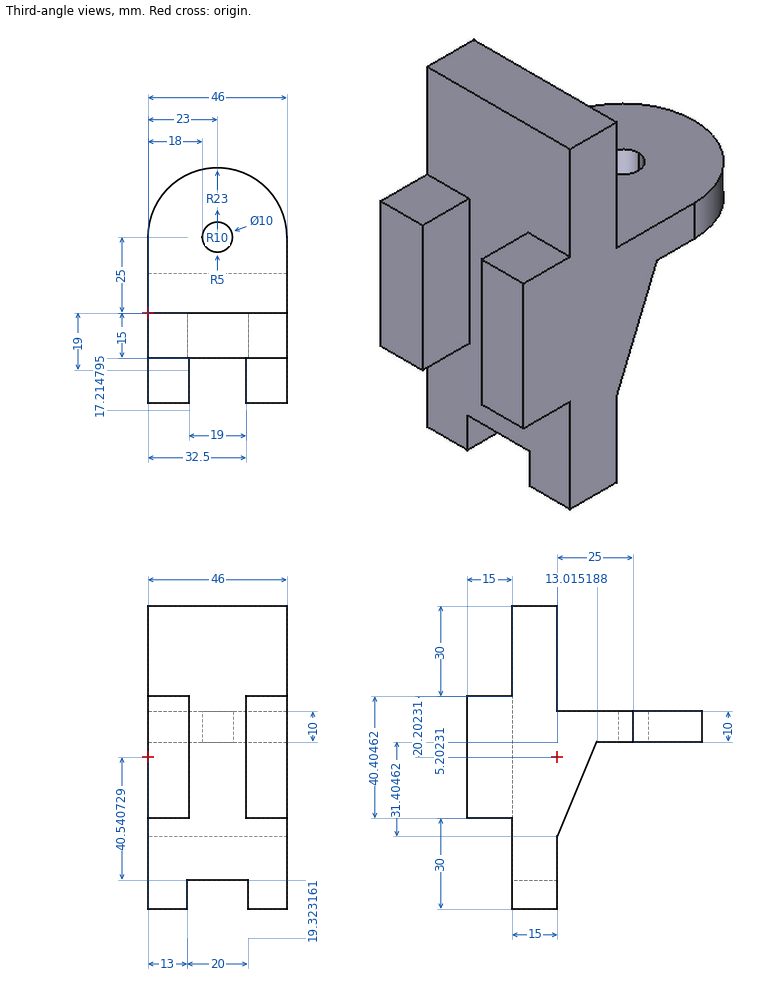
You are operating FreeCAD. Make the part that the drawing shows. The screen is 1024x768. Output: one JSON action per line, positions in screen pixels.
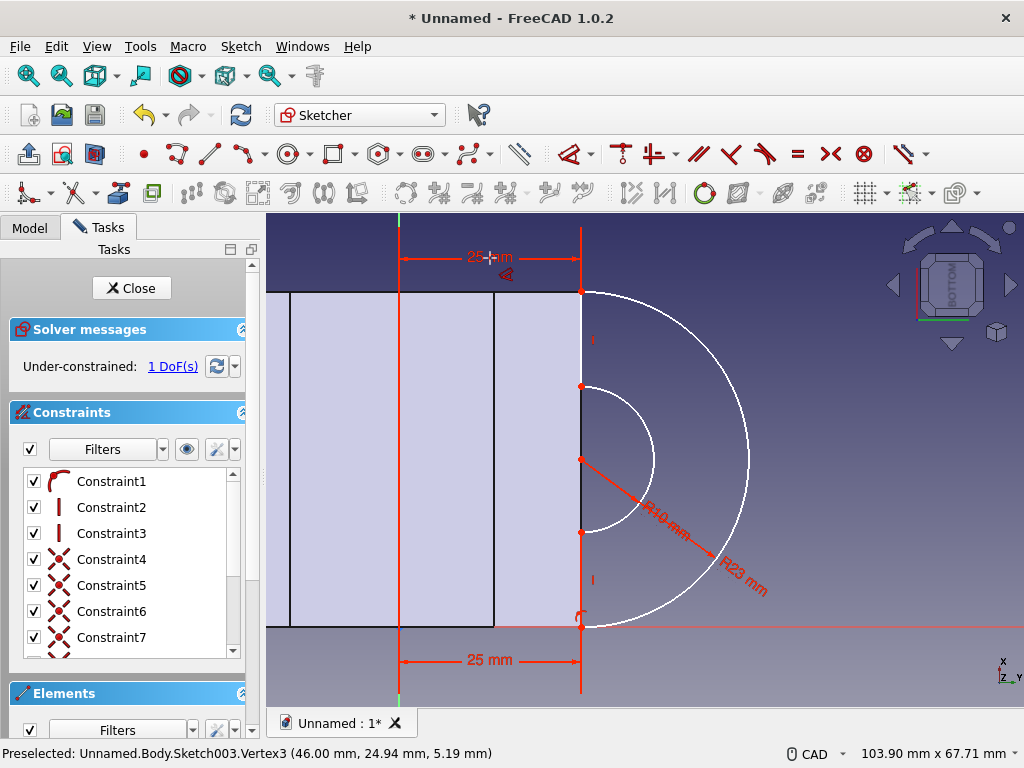
{"action": "left_click", "coordinate": [581, 460]}
{"action": "left_click", "coordinate": [490, 426]}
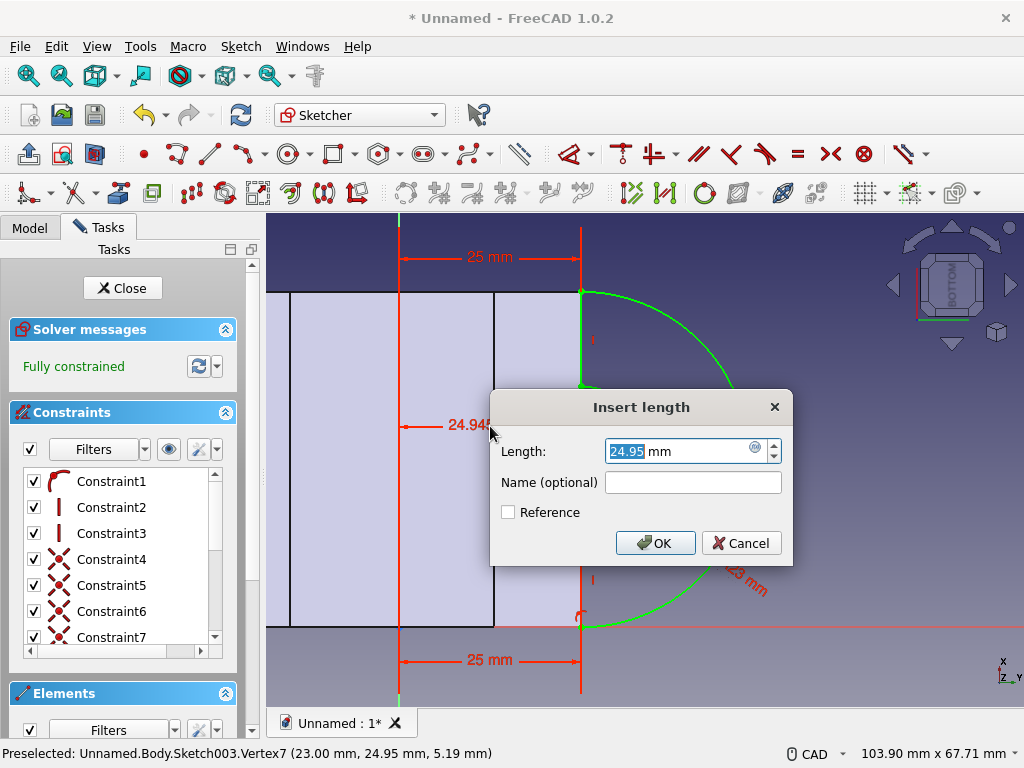
{"action": "type", "text": "25"}
{"action": "key", "text": "Return"}
{"action": "key", "text": "Escape"}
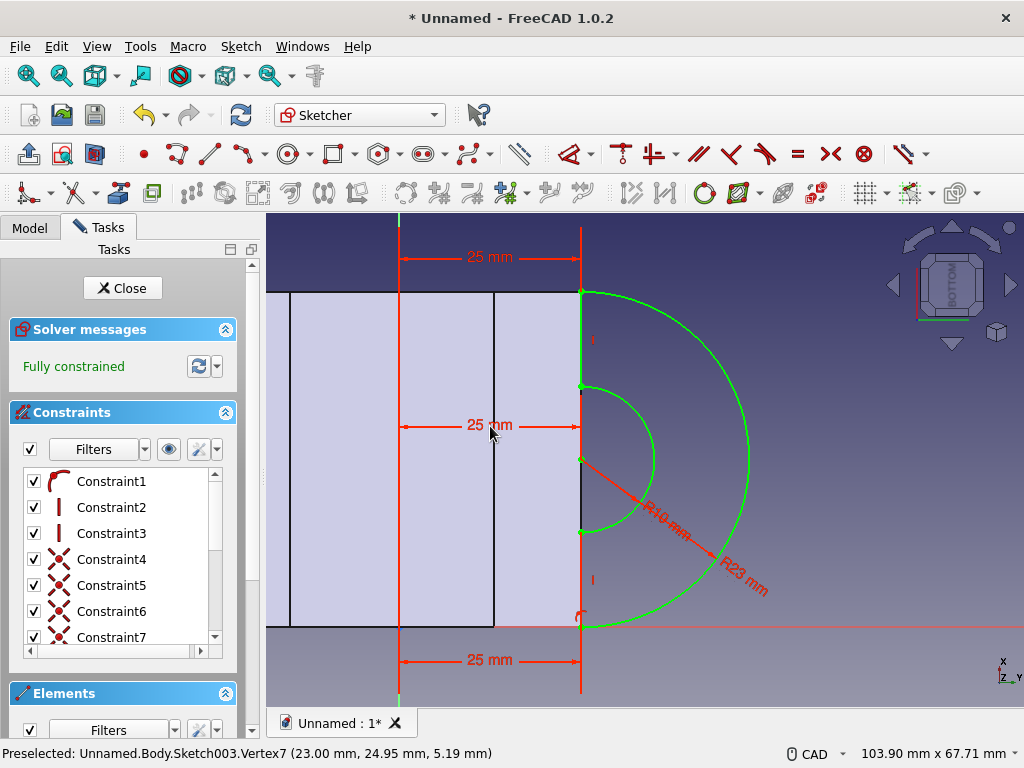
{"action": "left_click", "coordinate": [123, 288]}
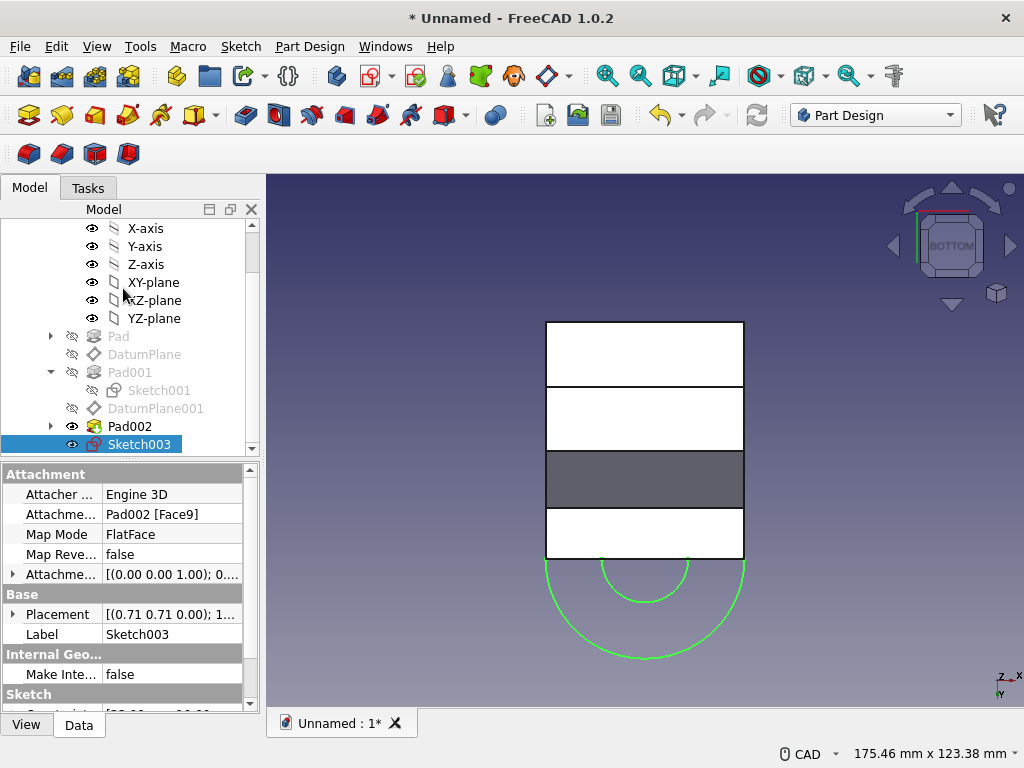
{"action": "left_click", "coordinate": [29, 116]}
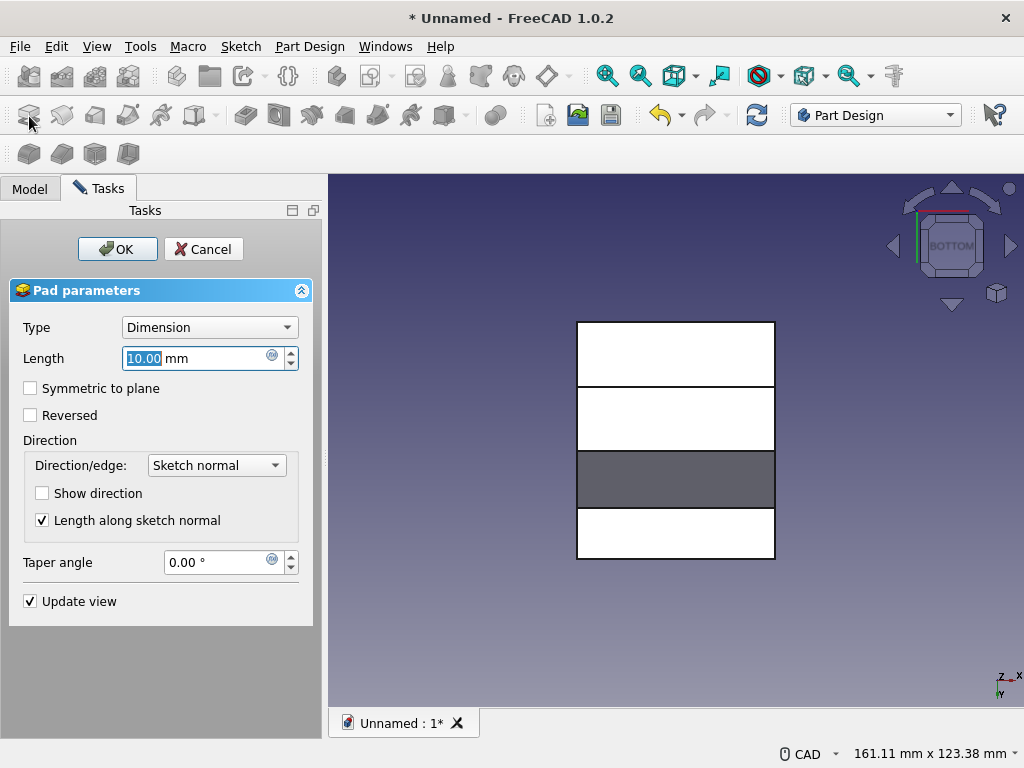
{"action": "type", "text": "10"}
{"action": "key", "text": "Tab"}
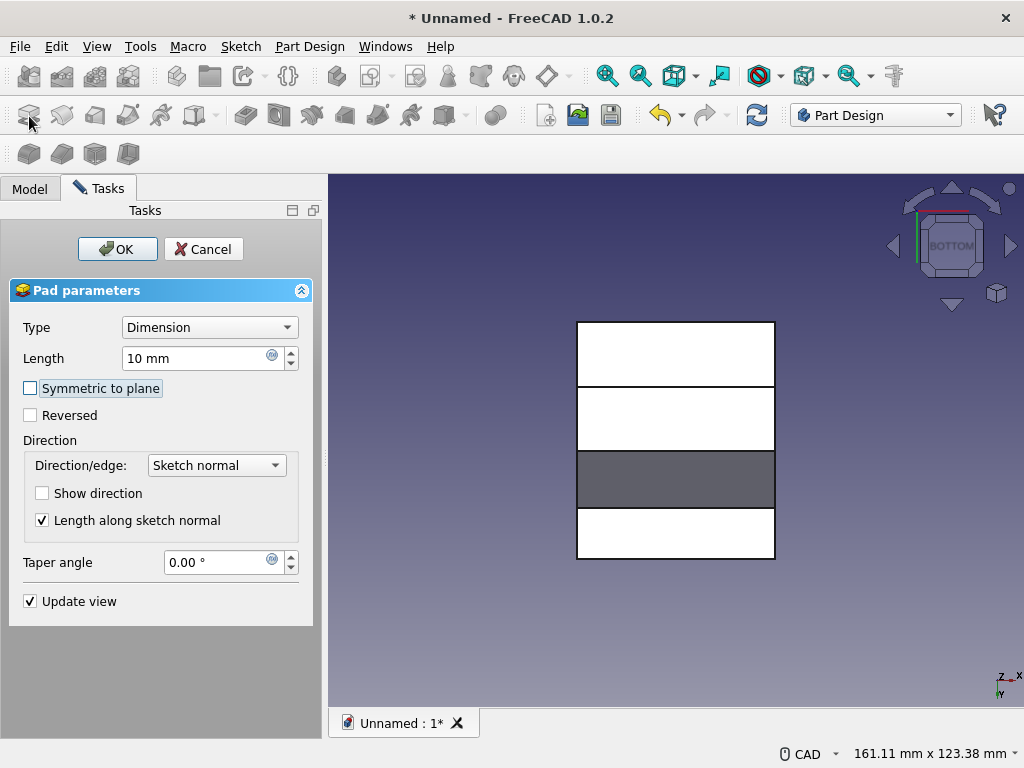
{"action": "left_click", "coordinate": [31, 415]}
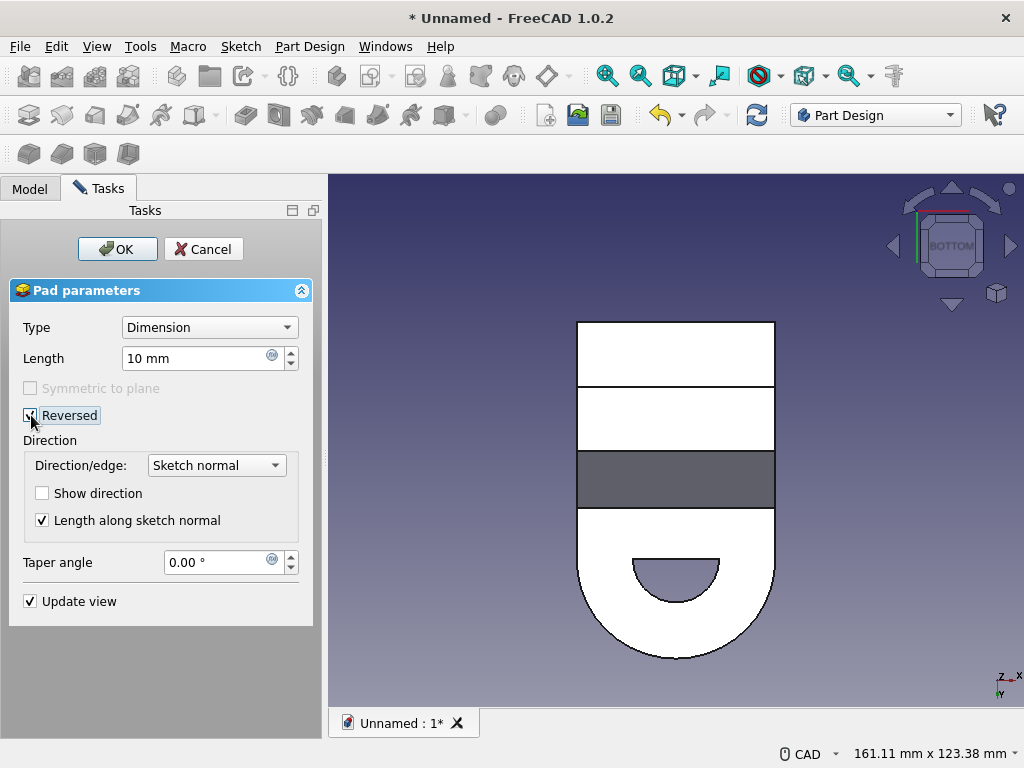
{"action": "left_click", "coordinate": [118, 249]}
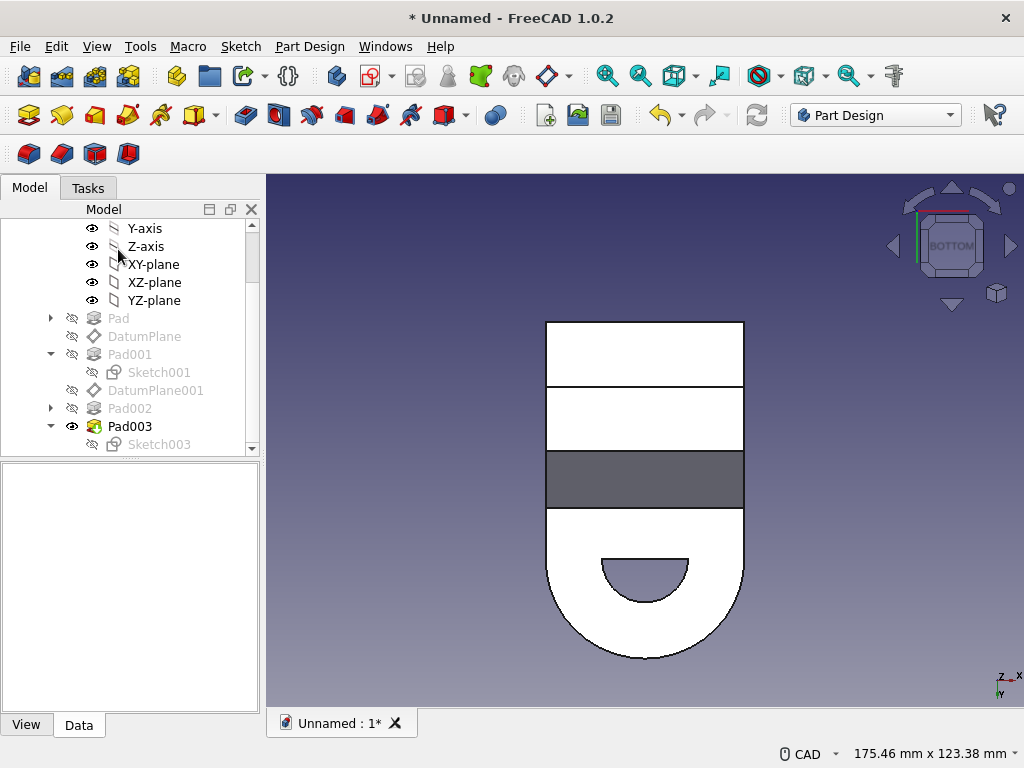
{"action": "left_click", "coordinate": [588, 604]}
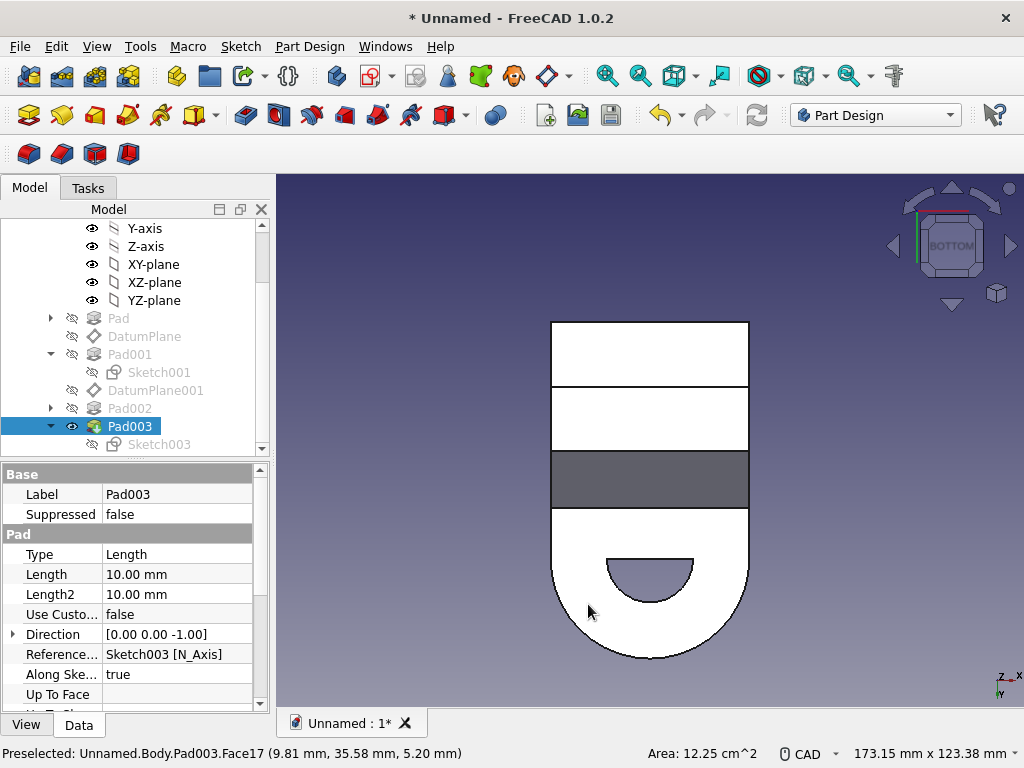
{"action": "left_click", "coordinate": [370, 76]}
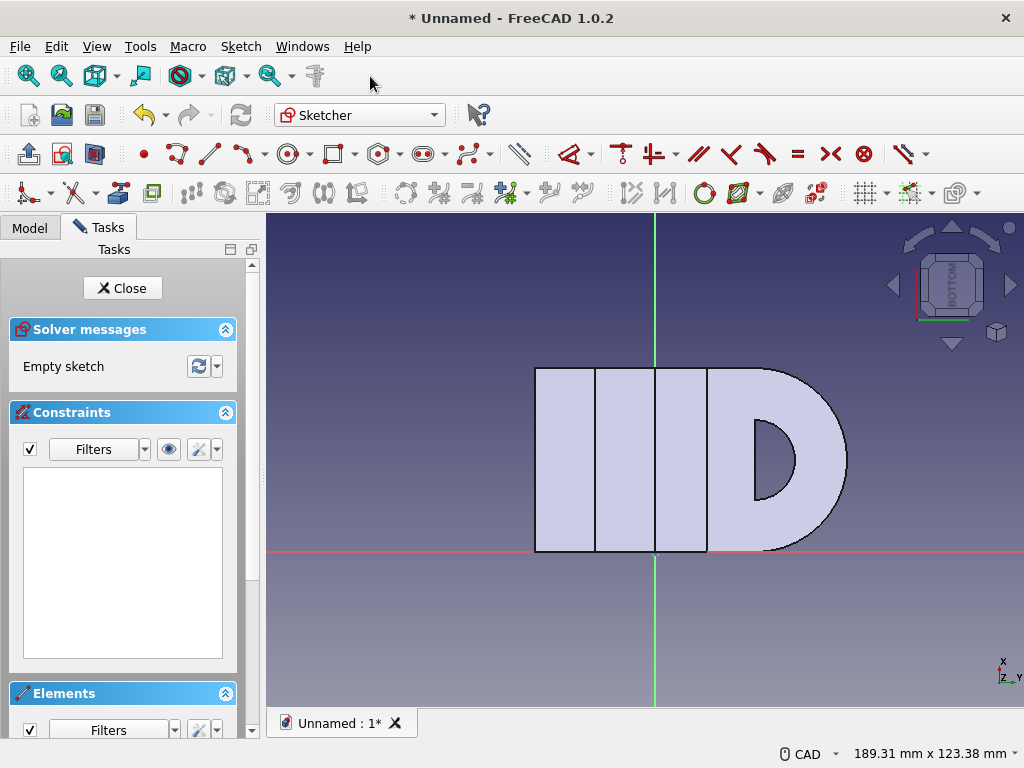
{"action": "scroll", "coordinate": [846, 507], "scroll_direction": "up", "scroll_amount": 4}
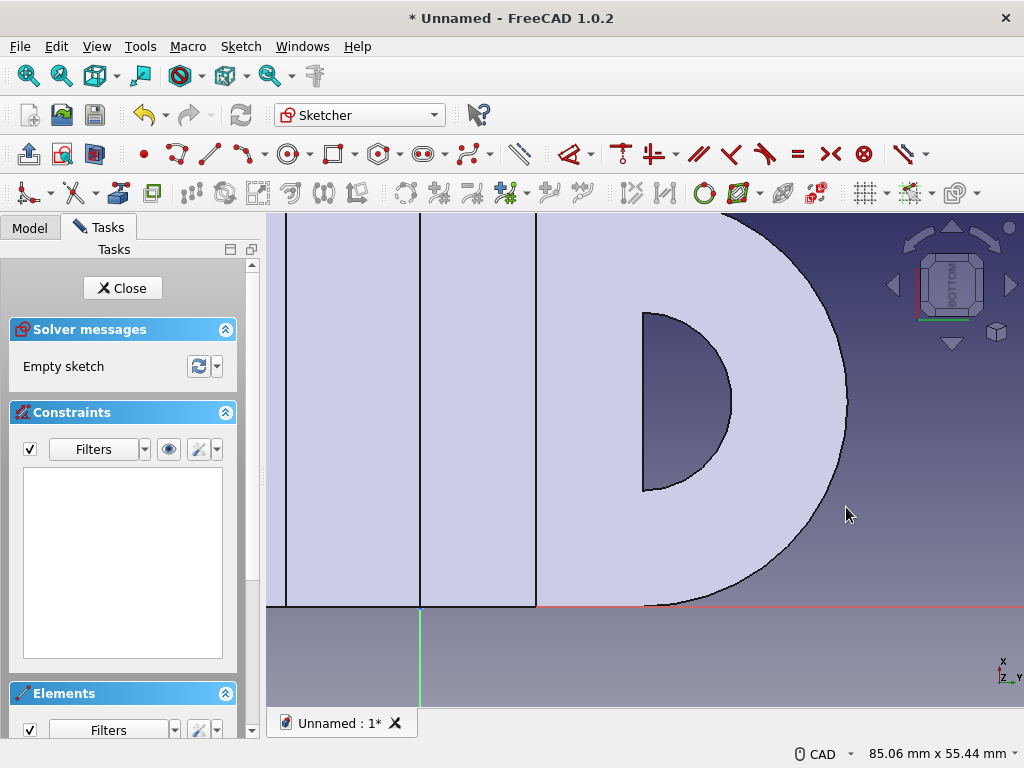
{"action": "key", "text": "g l"}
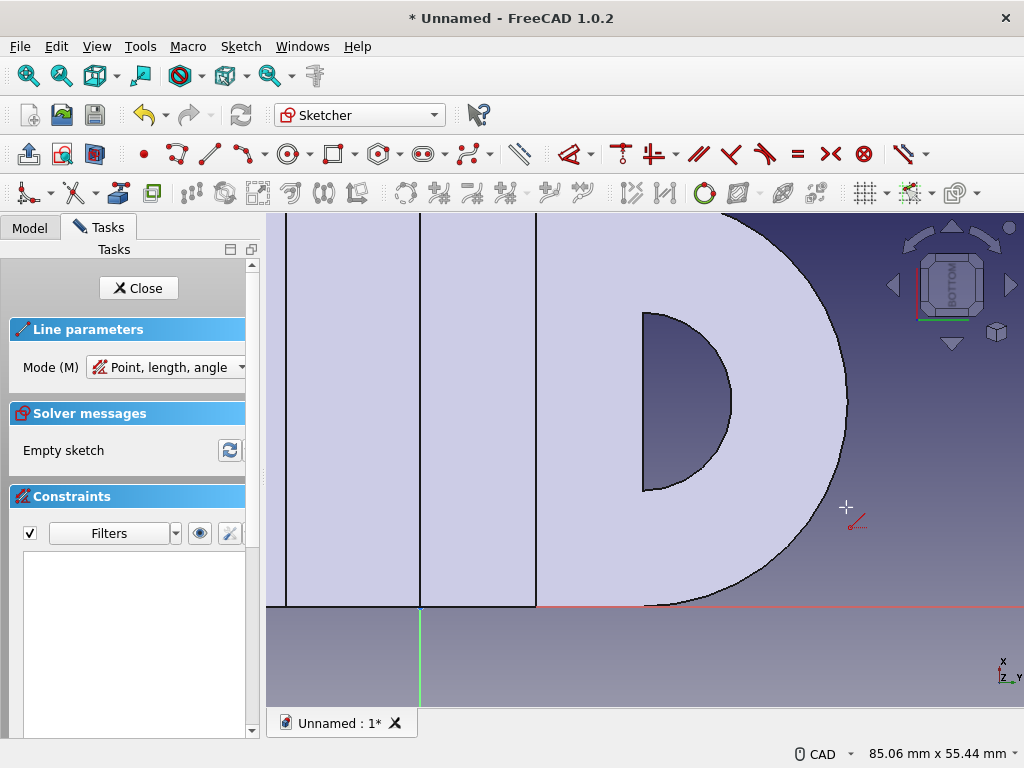
{"action": "left_click", "coordinate": [643, 446]}
{"action": "left_click", "coordinate": [643, 491]}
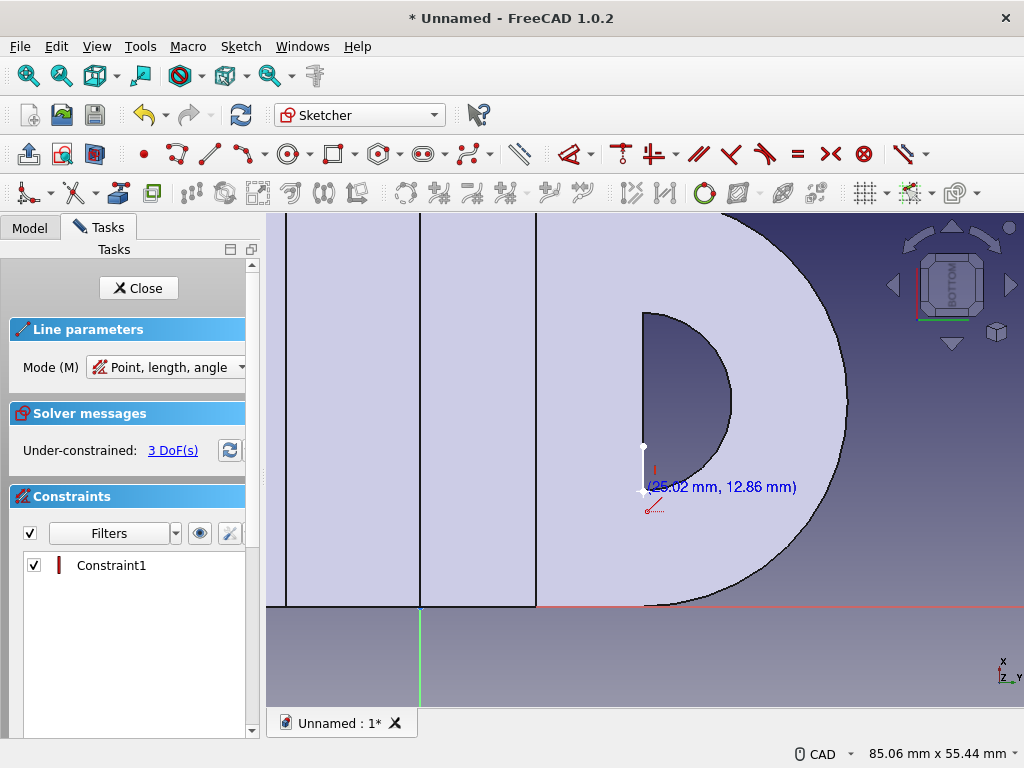
{"action": "left_click", "coordinate": [643, 313]}
{"action": "left_click", "coordinate": [643, 357]}